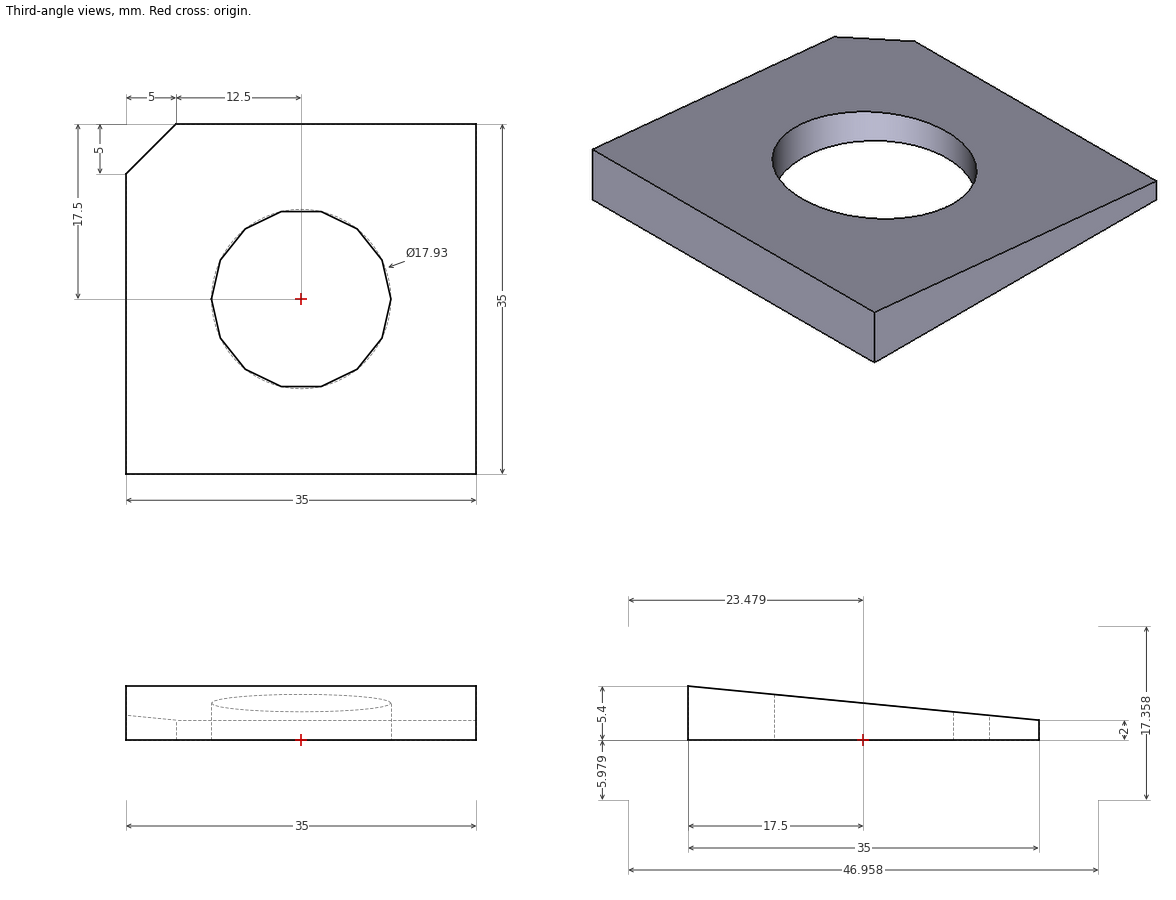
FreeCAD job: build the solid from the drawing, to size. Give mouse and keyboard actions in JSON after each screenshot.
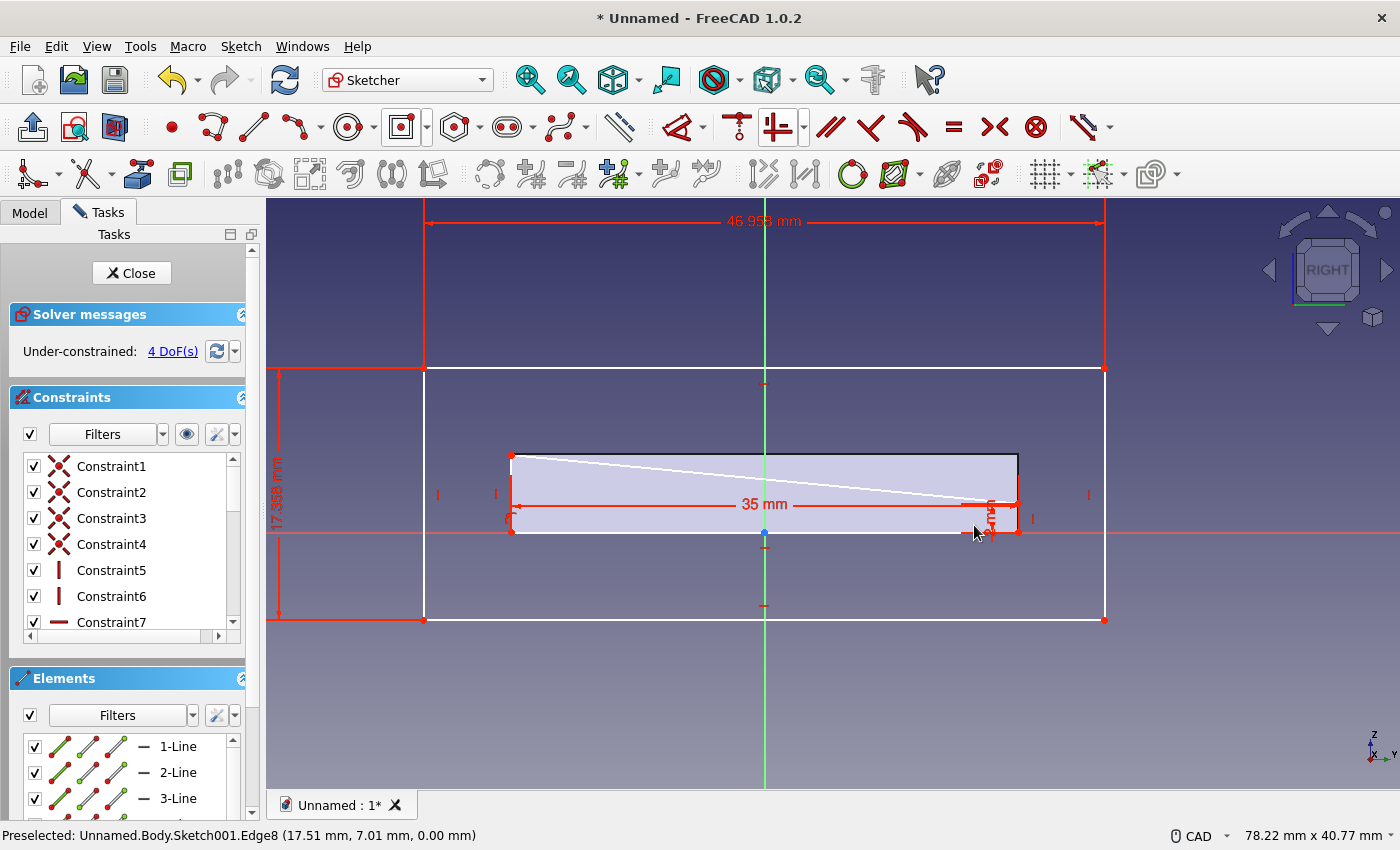
{"action": "left_click", "coordinate": [511, 509]}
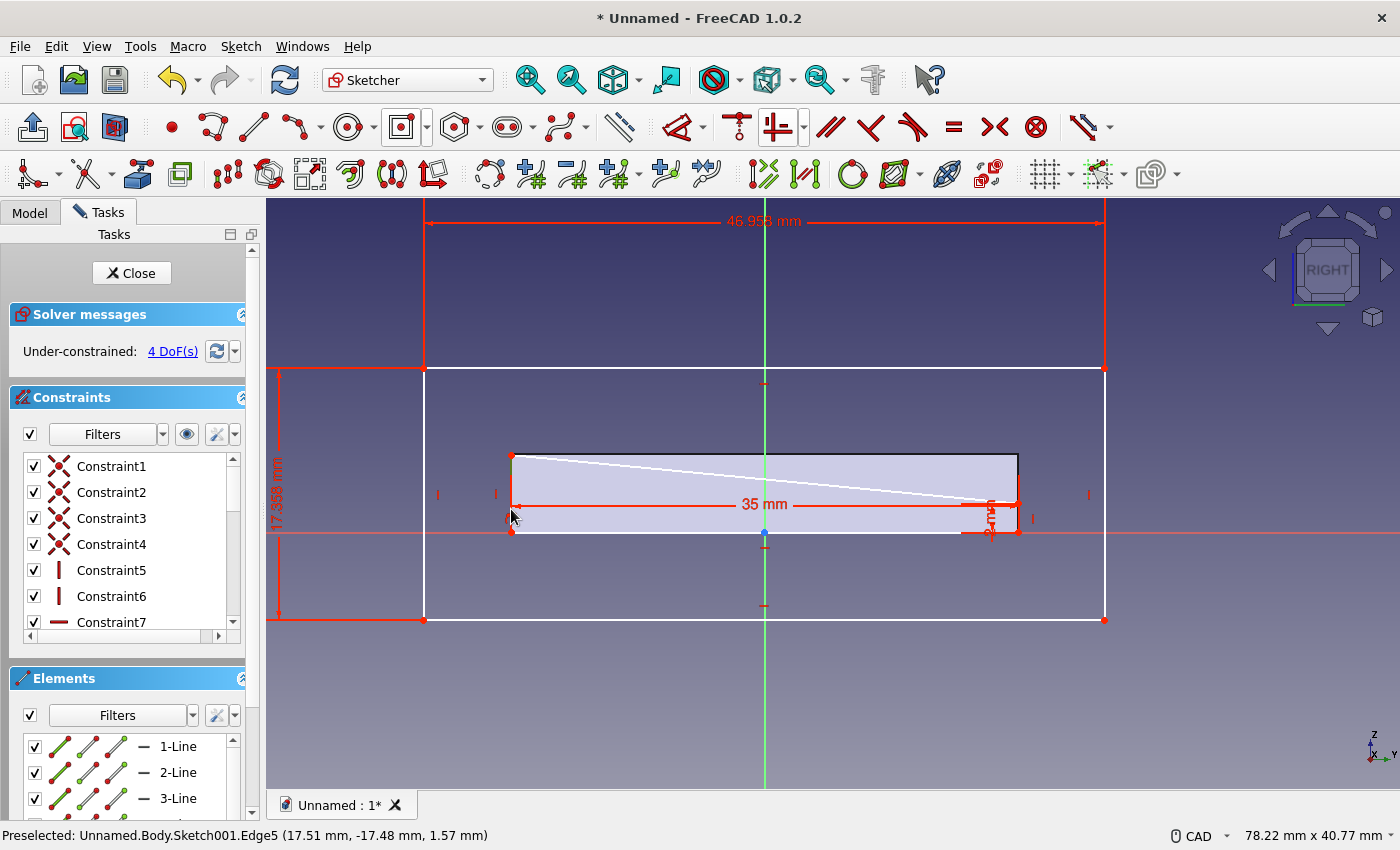
{"action": "key", "text": "i"}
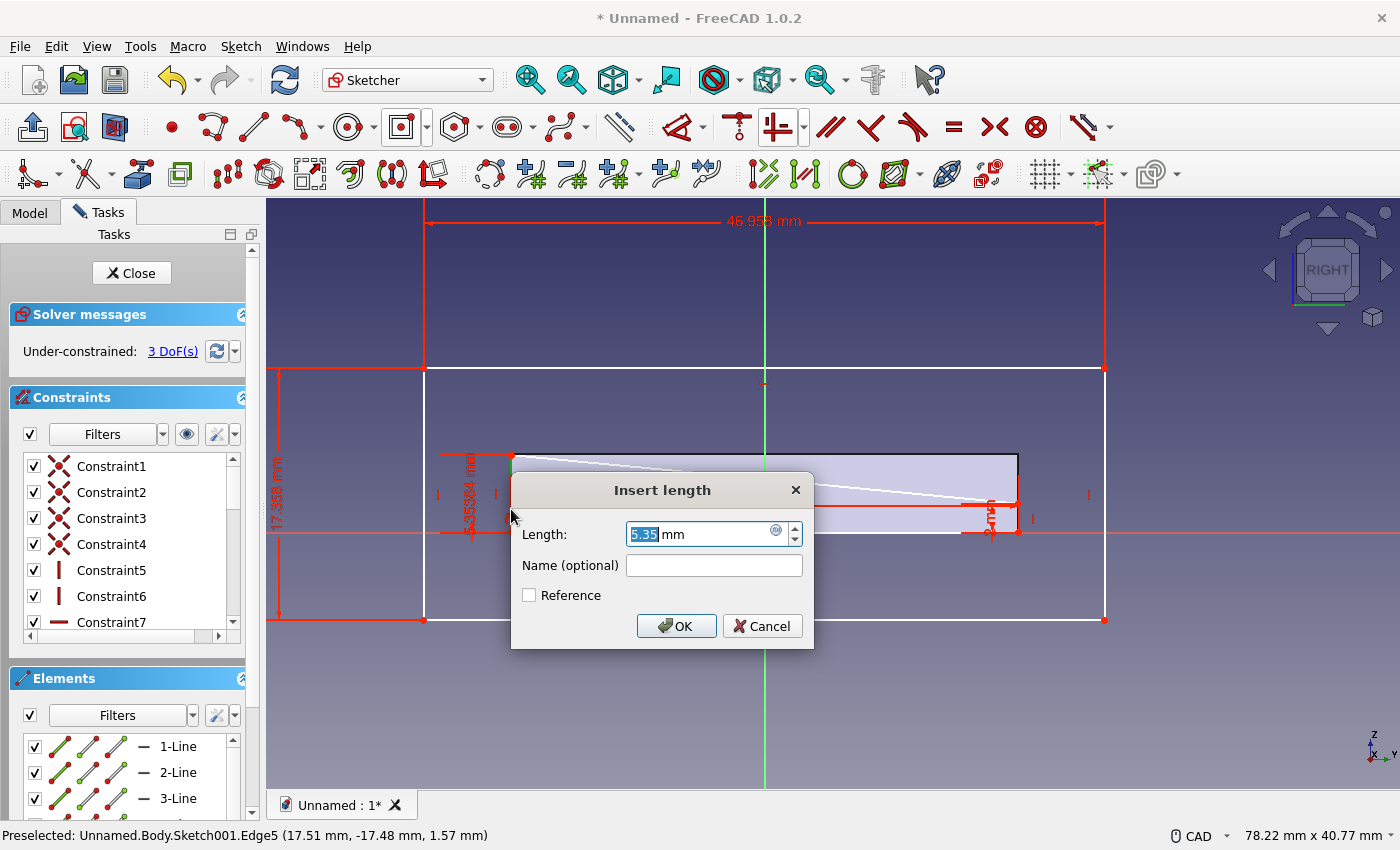
{"action": "type", "text": "5.4"}
{"action": "key", "text": "Return"}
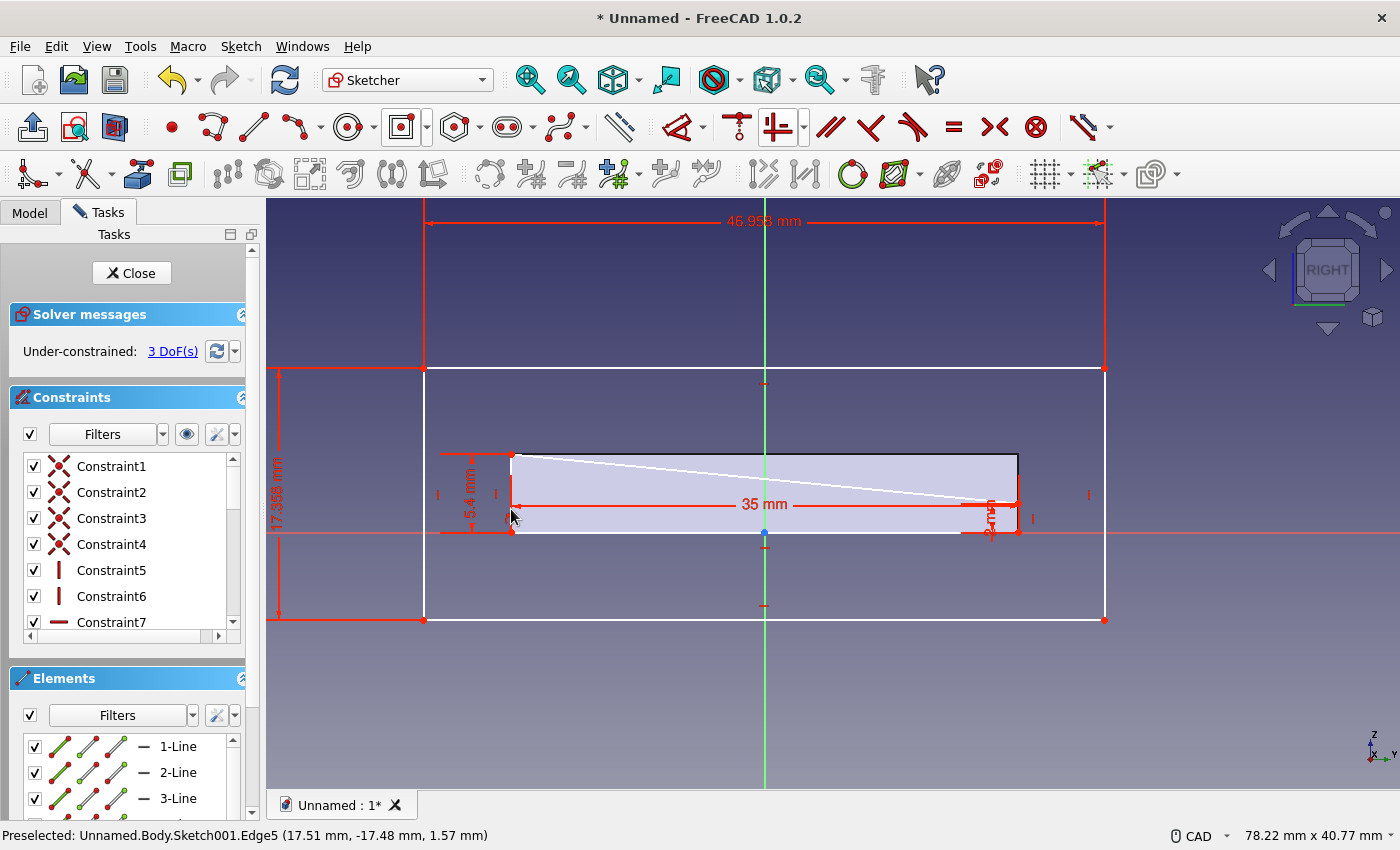
{"action": "left_click", "coordinate": [511, 533]}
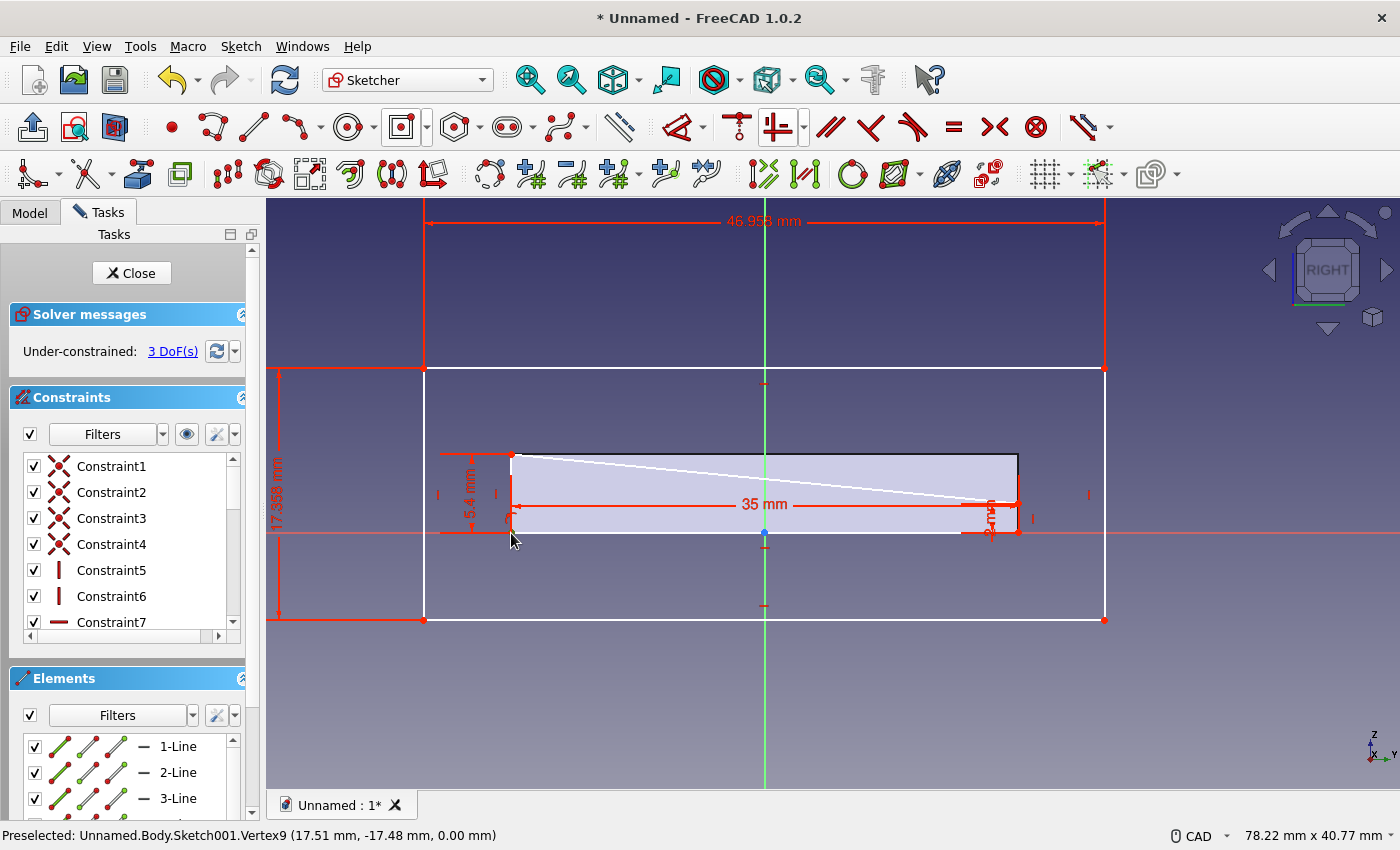
{"action": "key", "text": "l"}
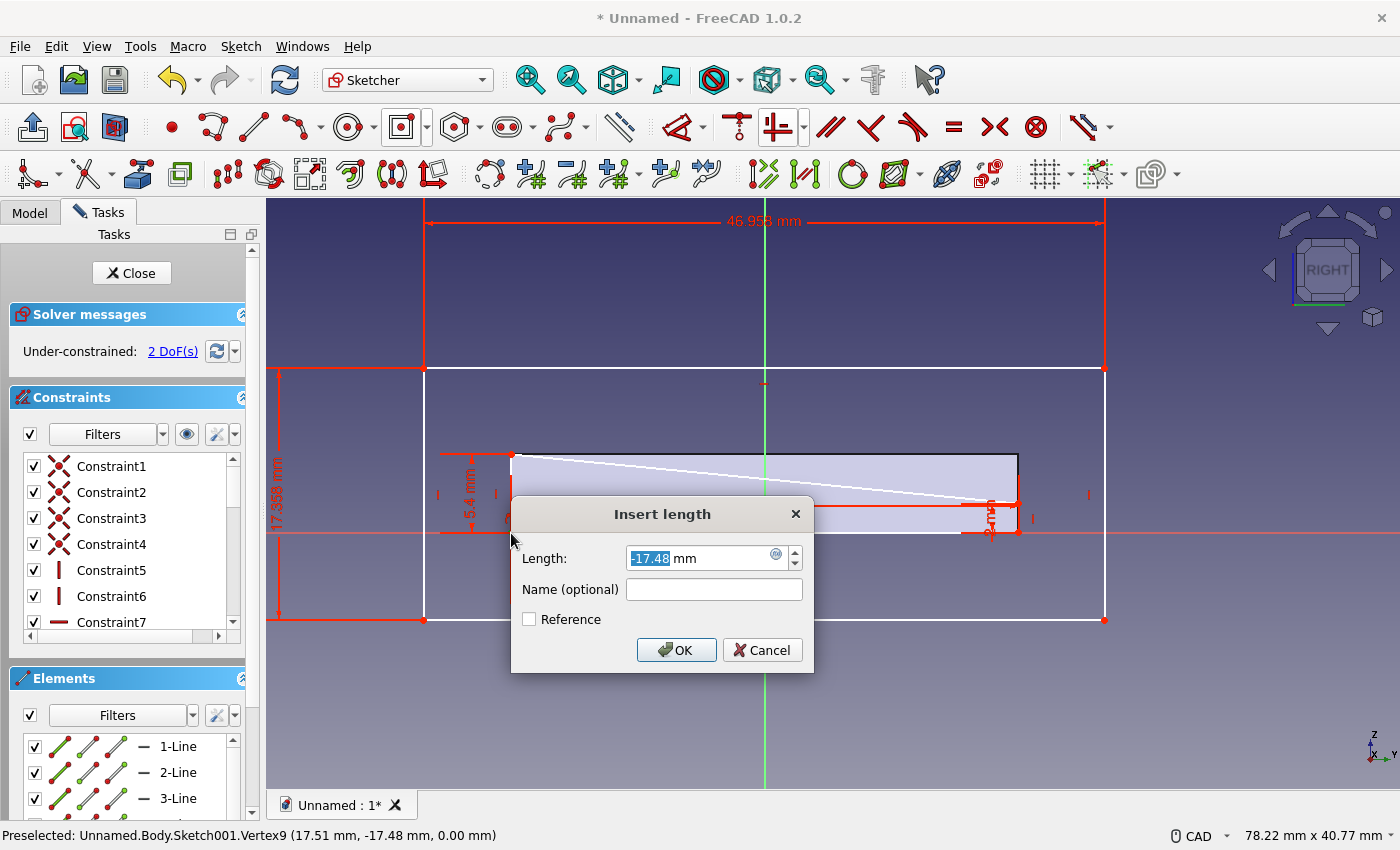
{"action": "type", "text": "-17.5"}
{"action": "key", "text": "Return"}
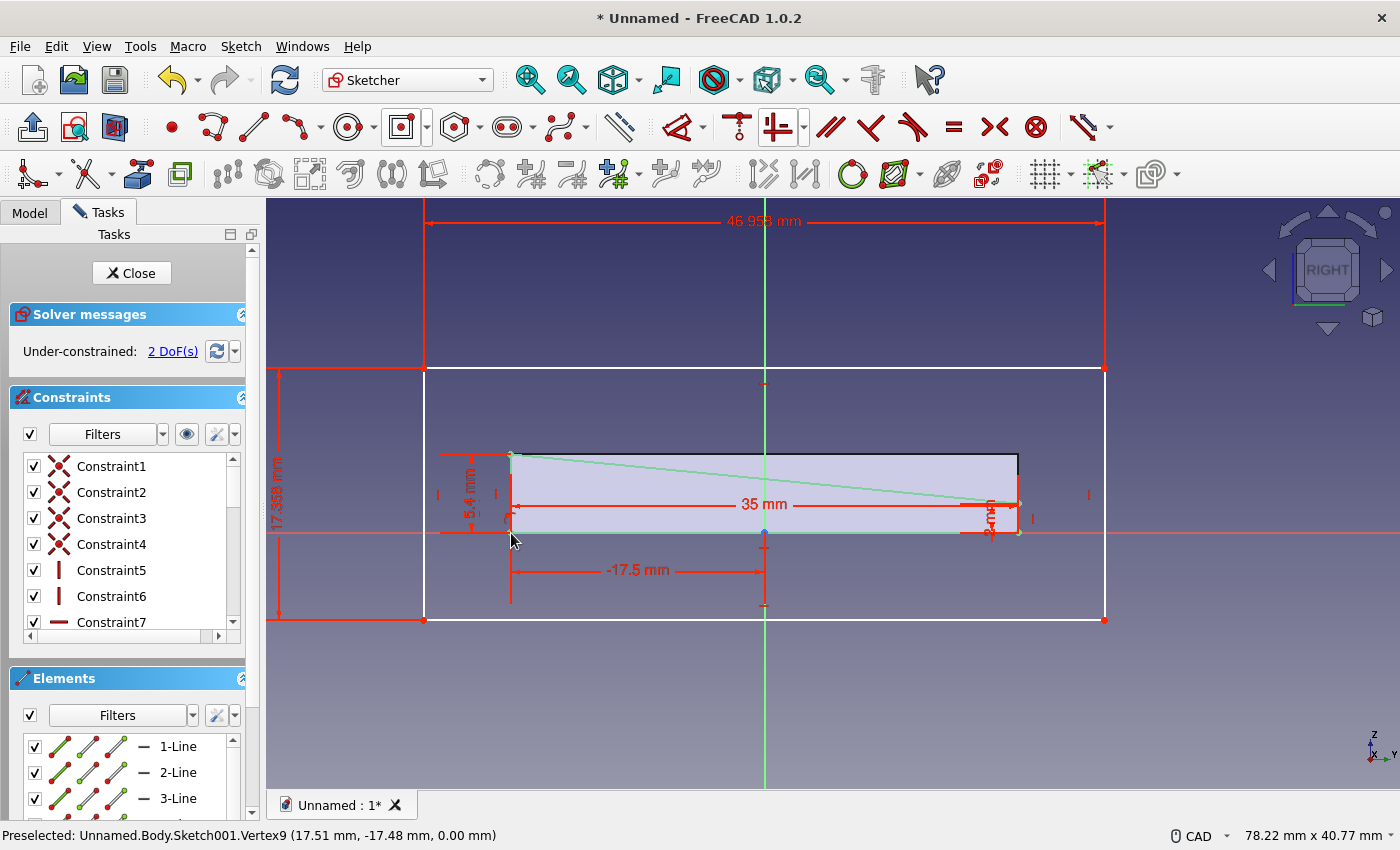
{"action": "left_click", "coordinate": [424, 620]}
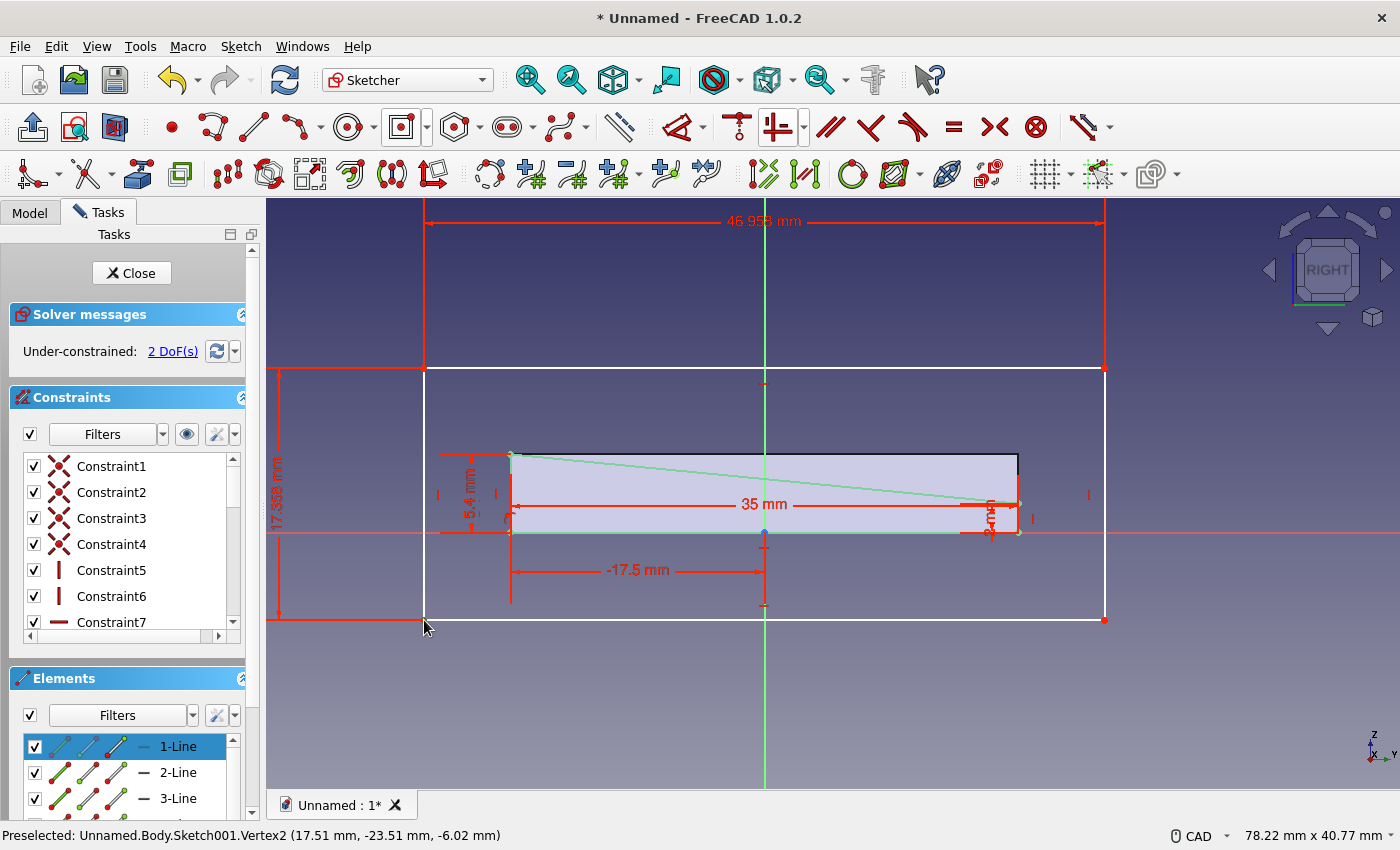
{"action": "key", "text": "i"}